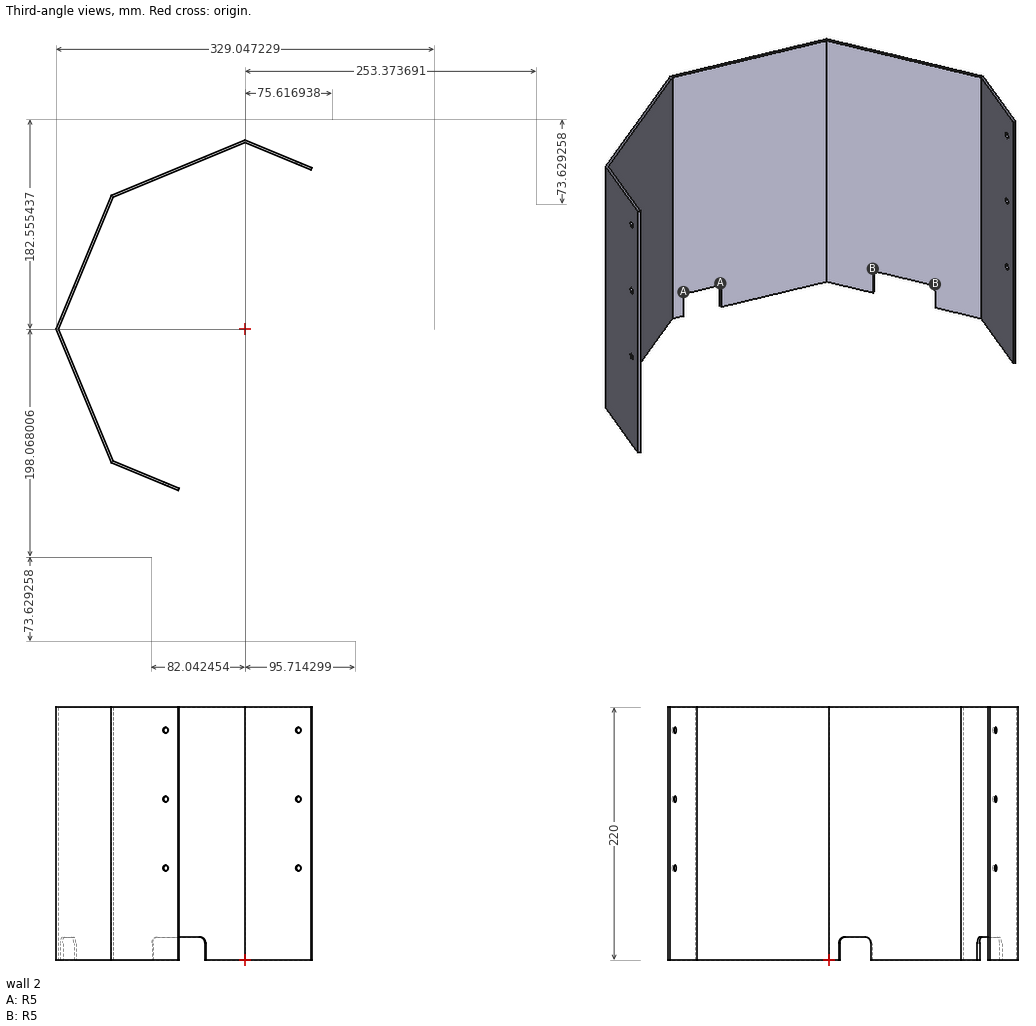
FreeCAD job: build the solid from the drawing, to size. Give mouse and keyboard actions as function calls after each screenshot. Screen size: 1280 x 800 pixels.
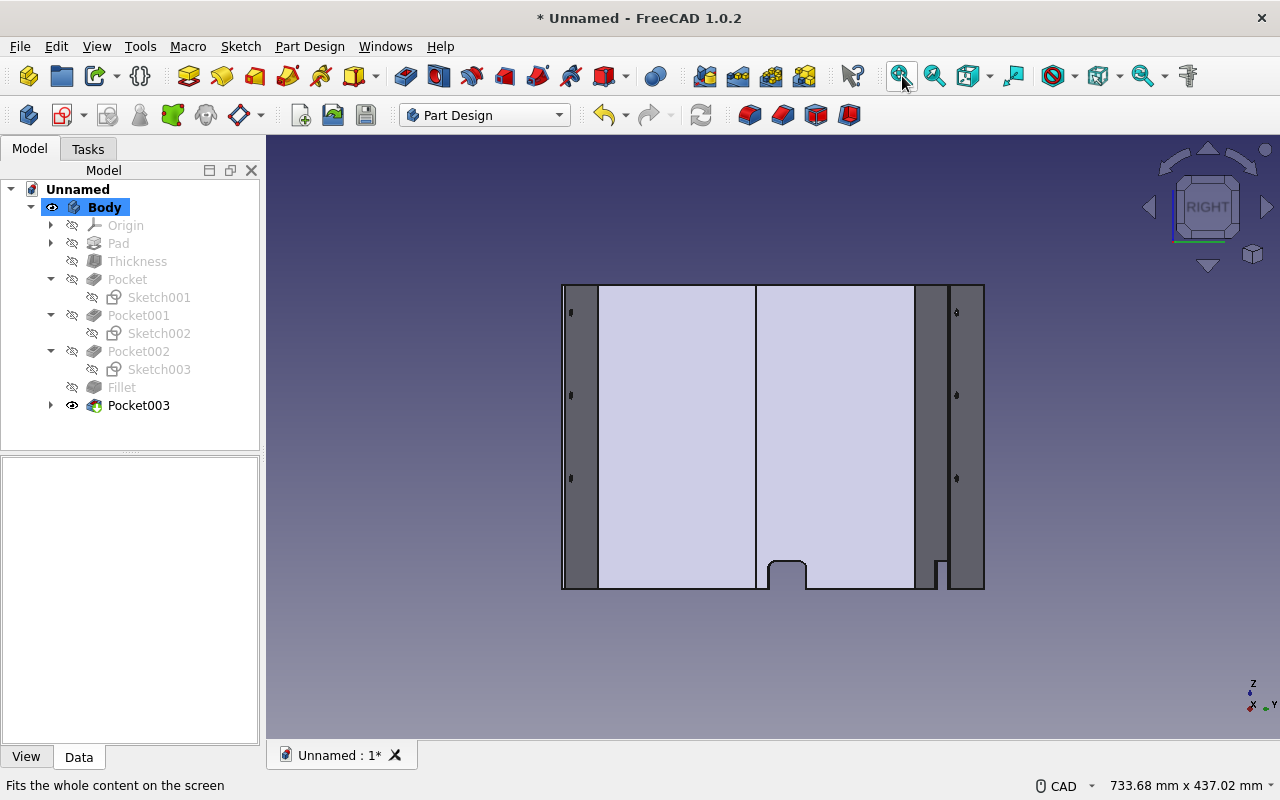
key(5)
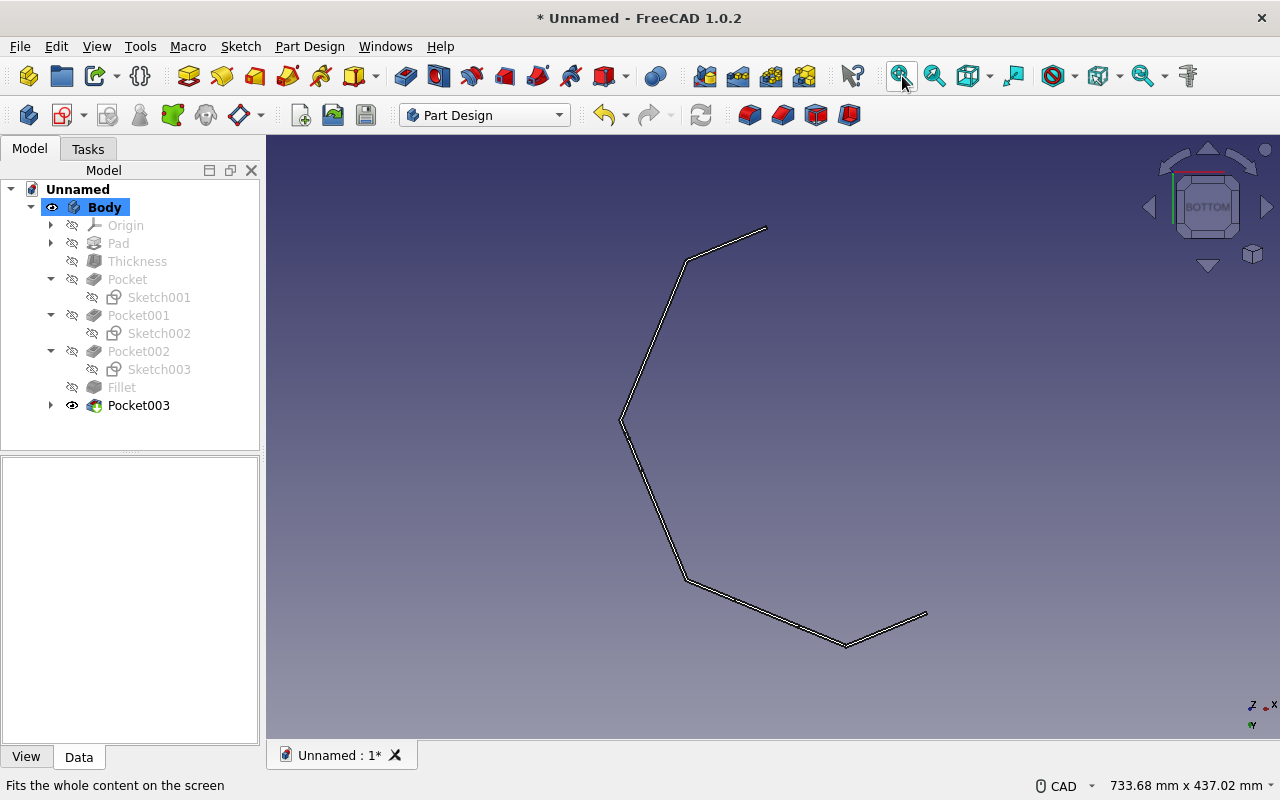
scroll(799, 625, up, 14)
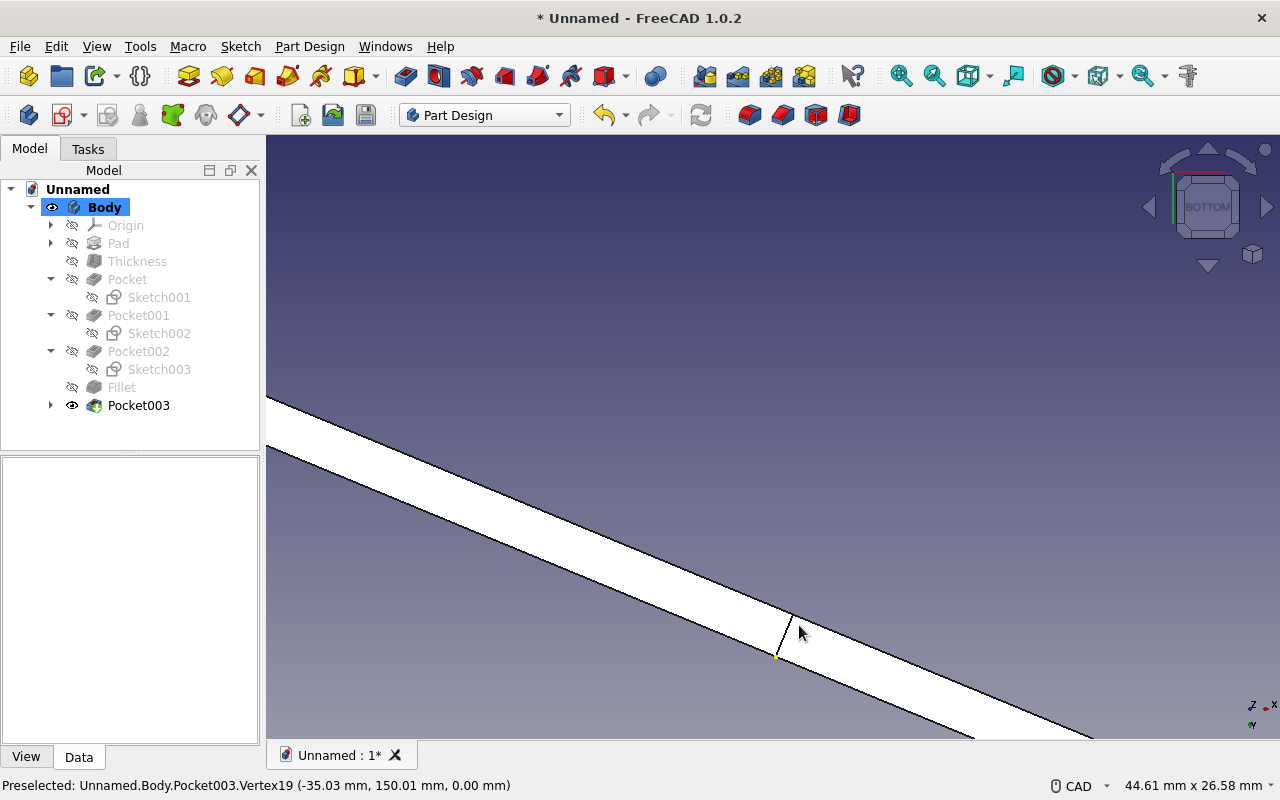
click(902, 76)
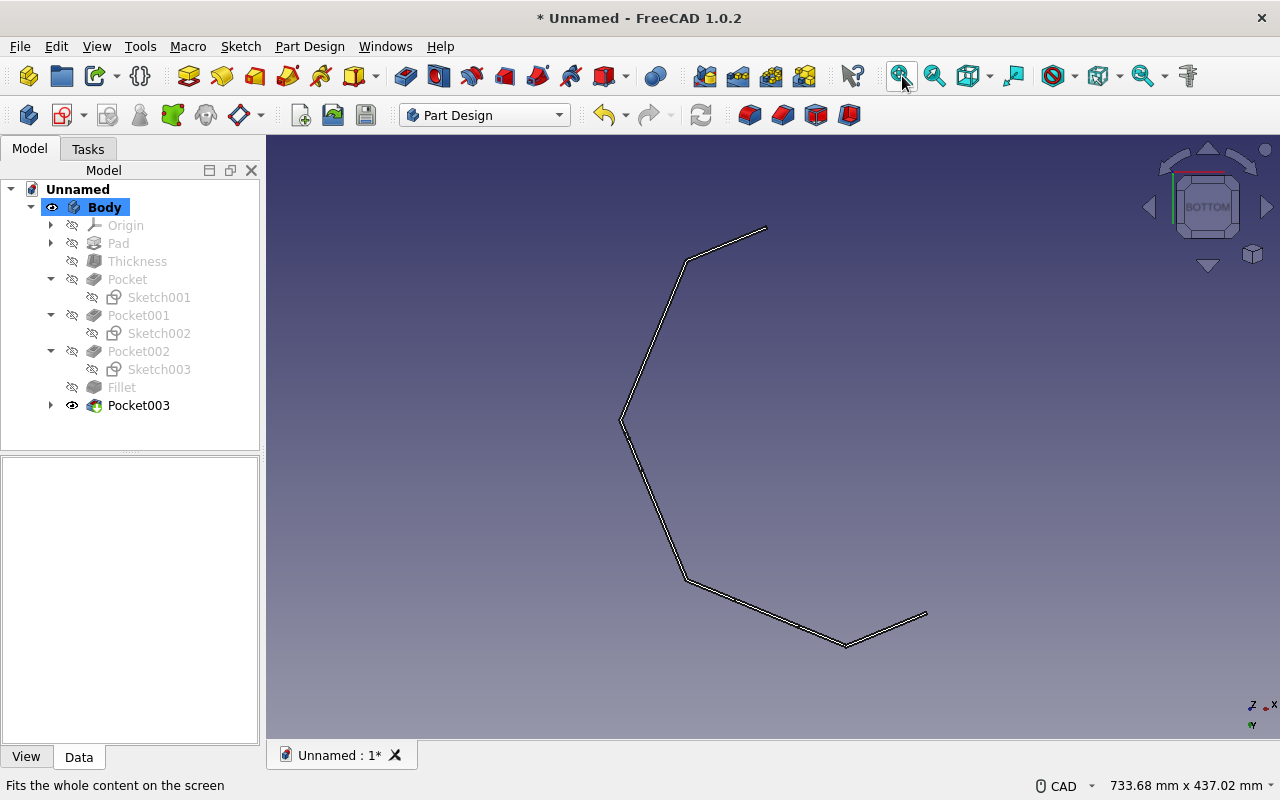
key(4)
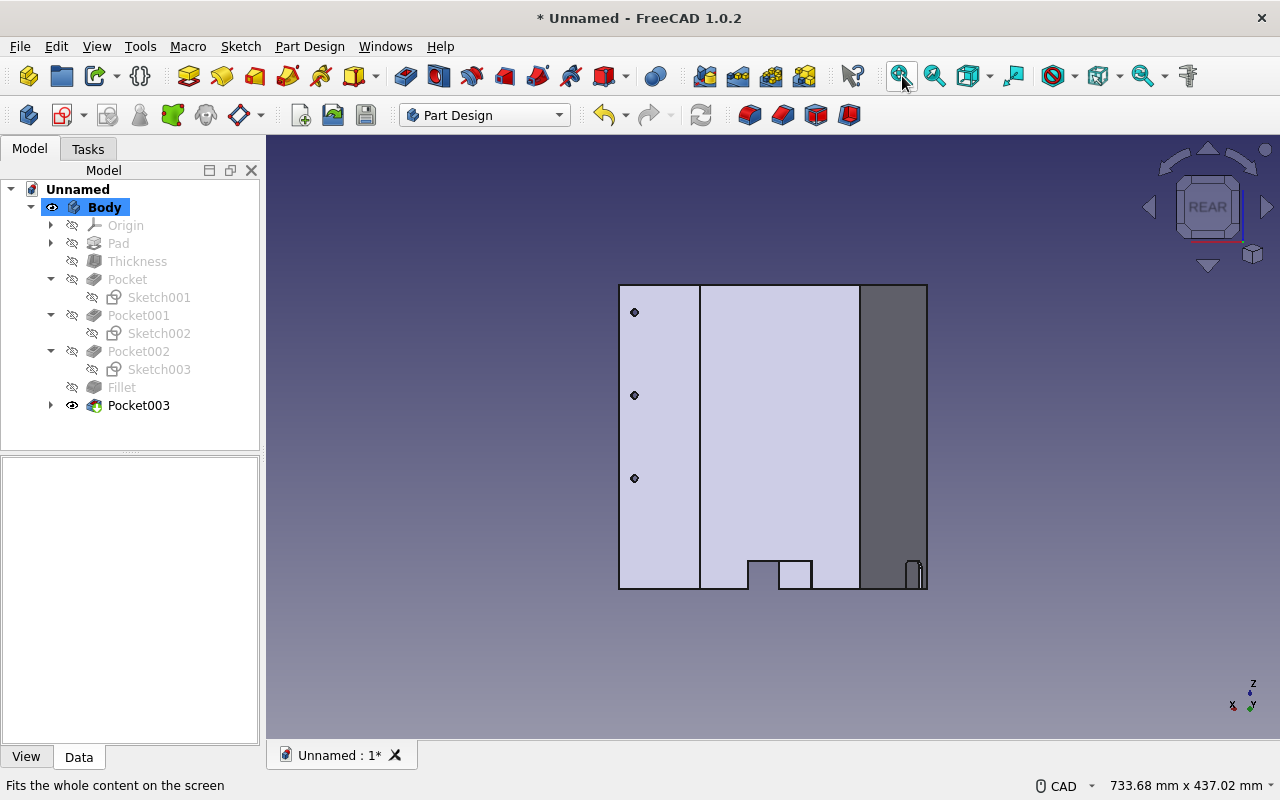
scroll(747, 560, up, 14)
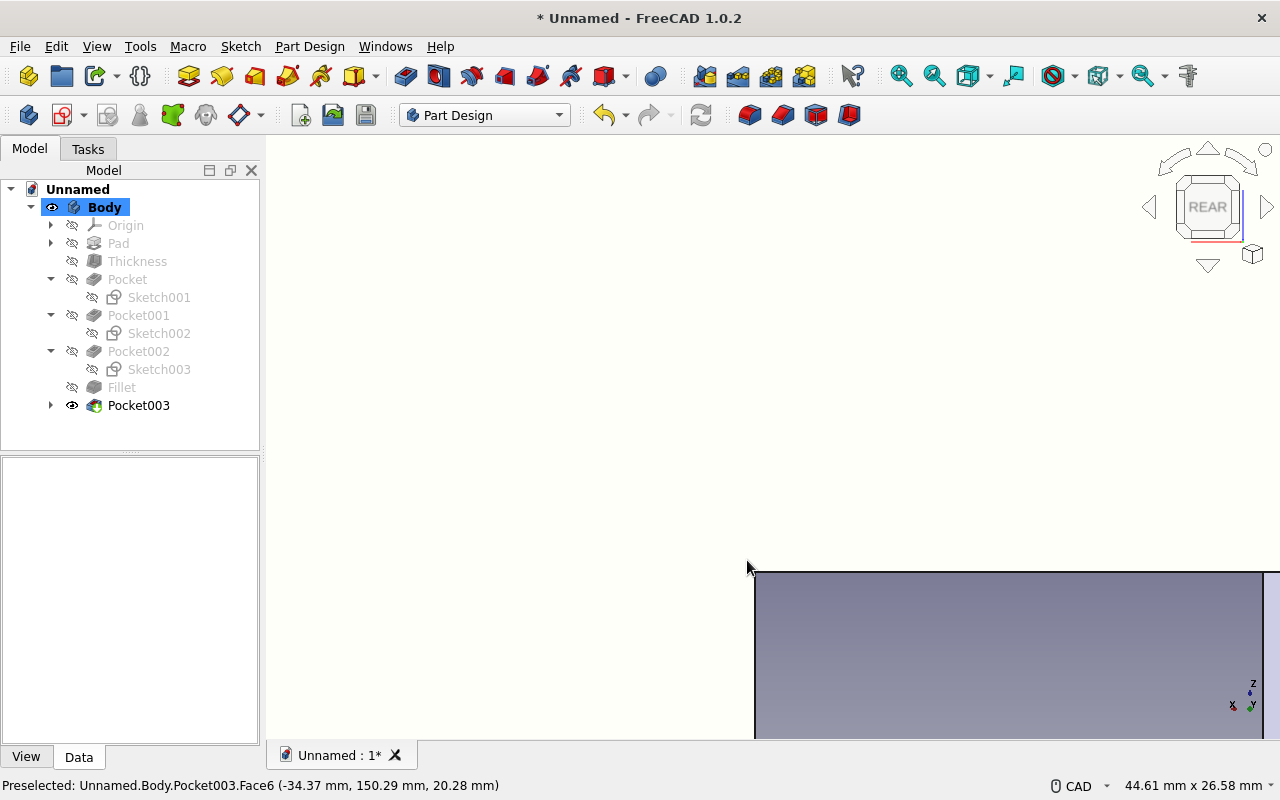
click(902, 76)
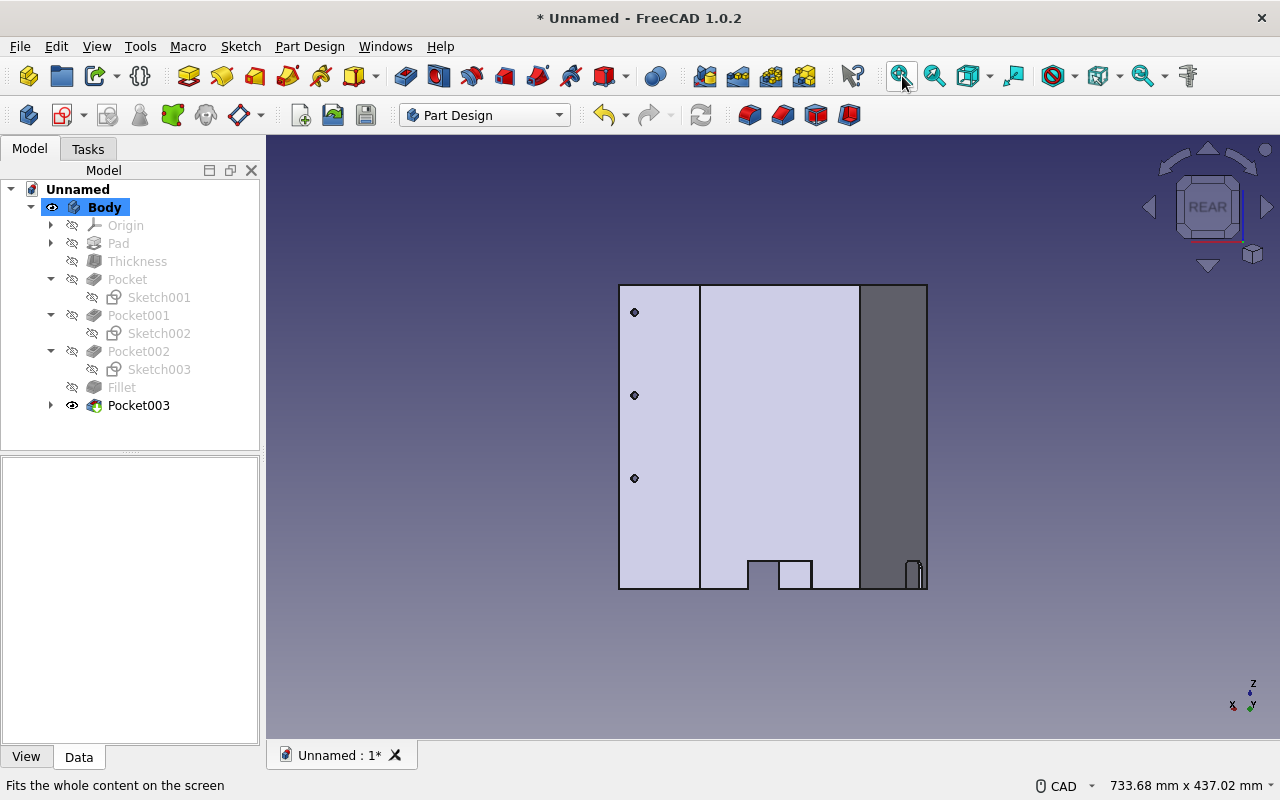
key(6)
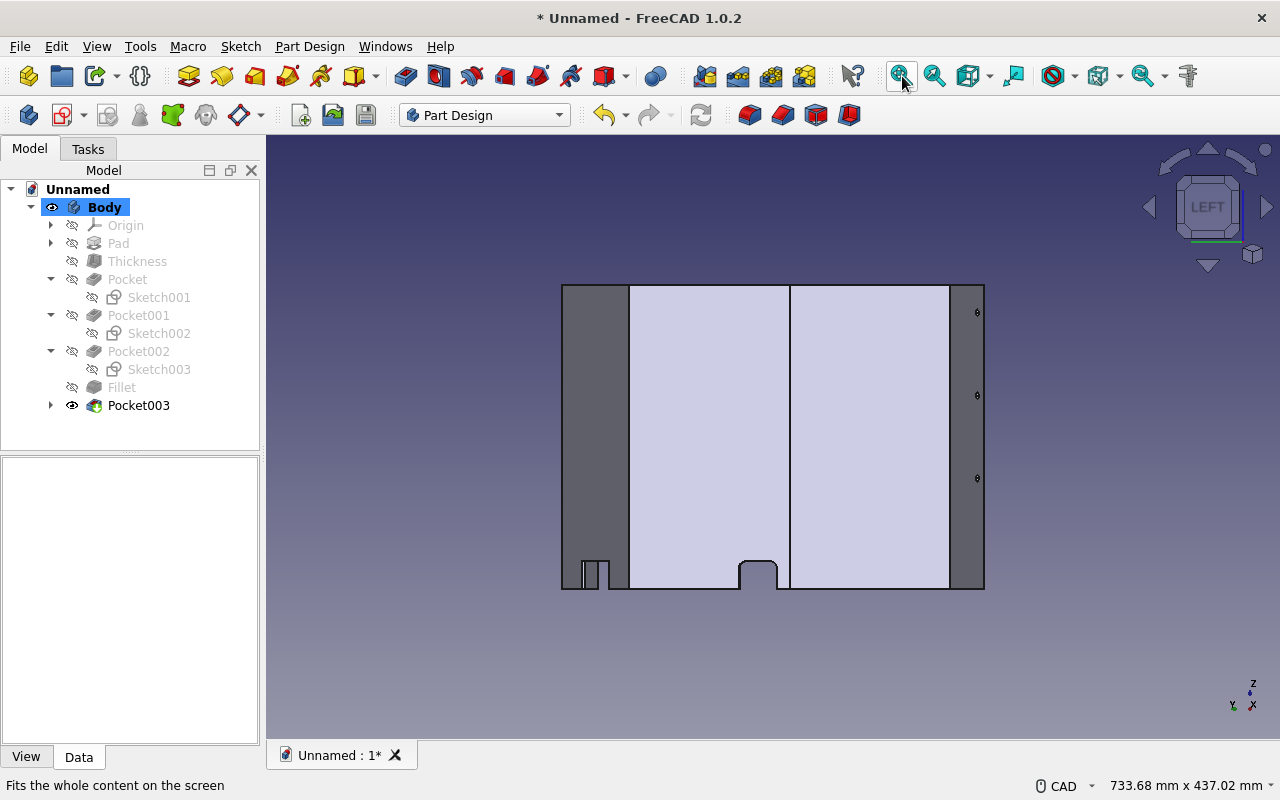
scroll(584, 560, up, 14)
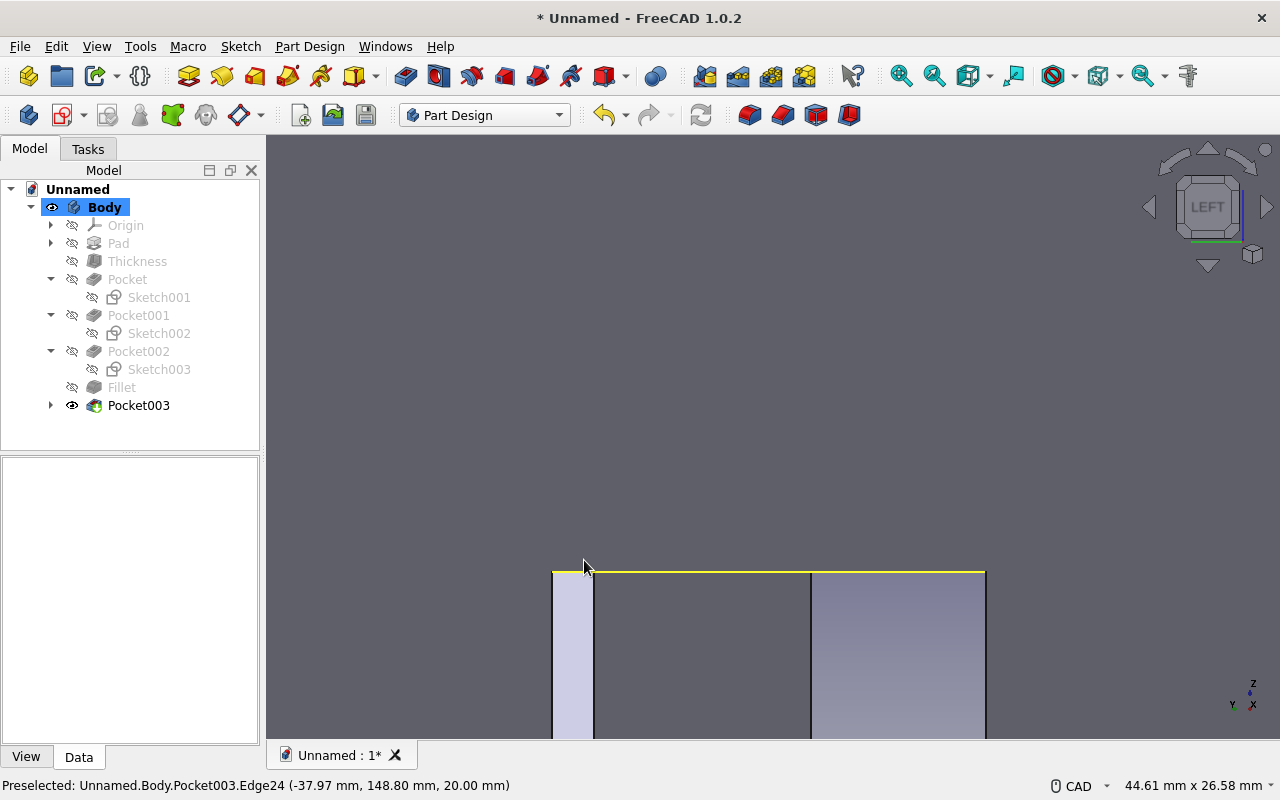
click(902, 76)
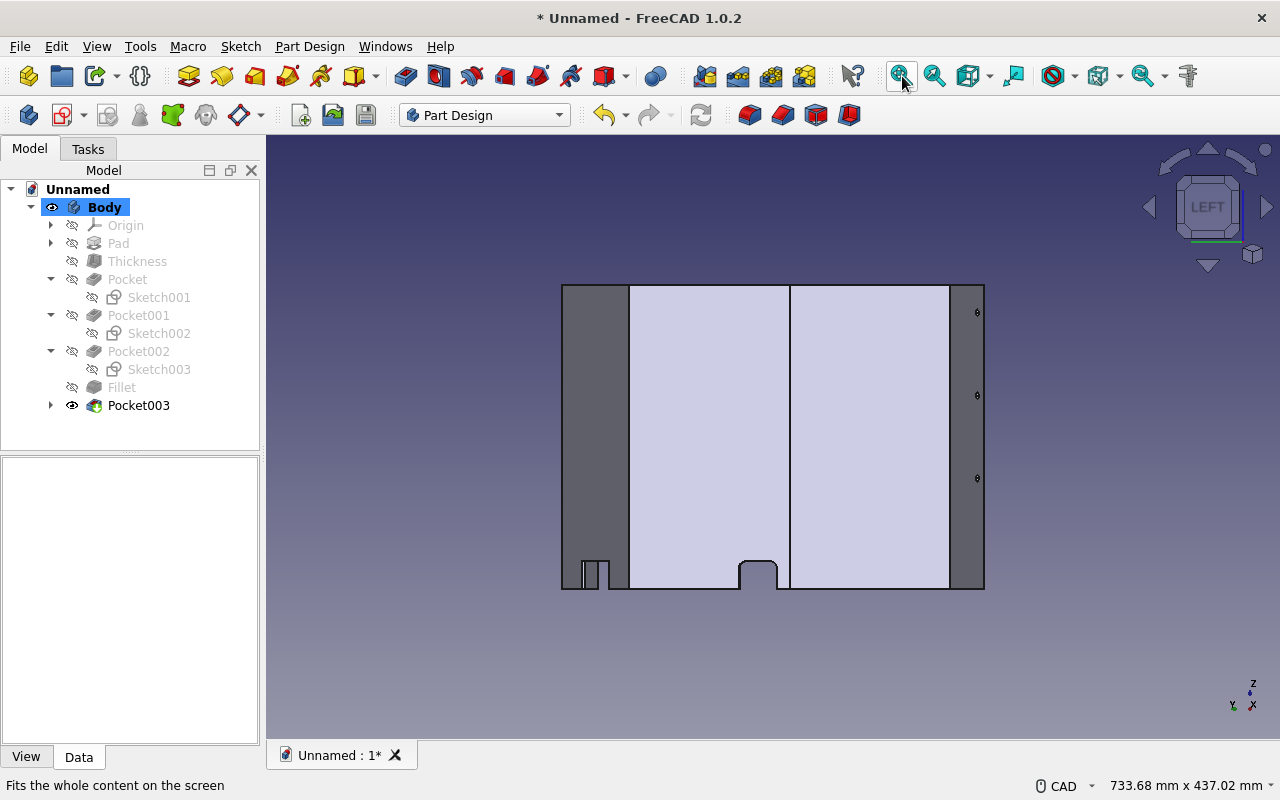
key(v)
key(3)